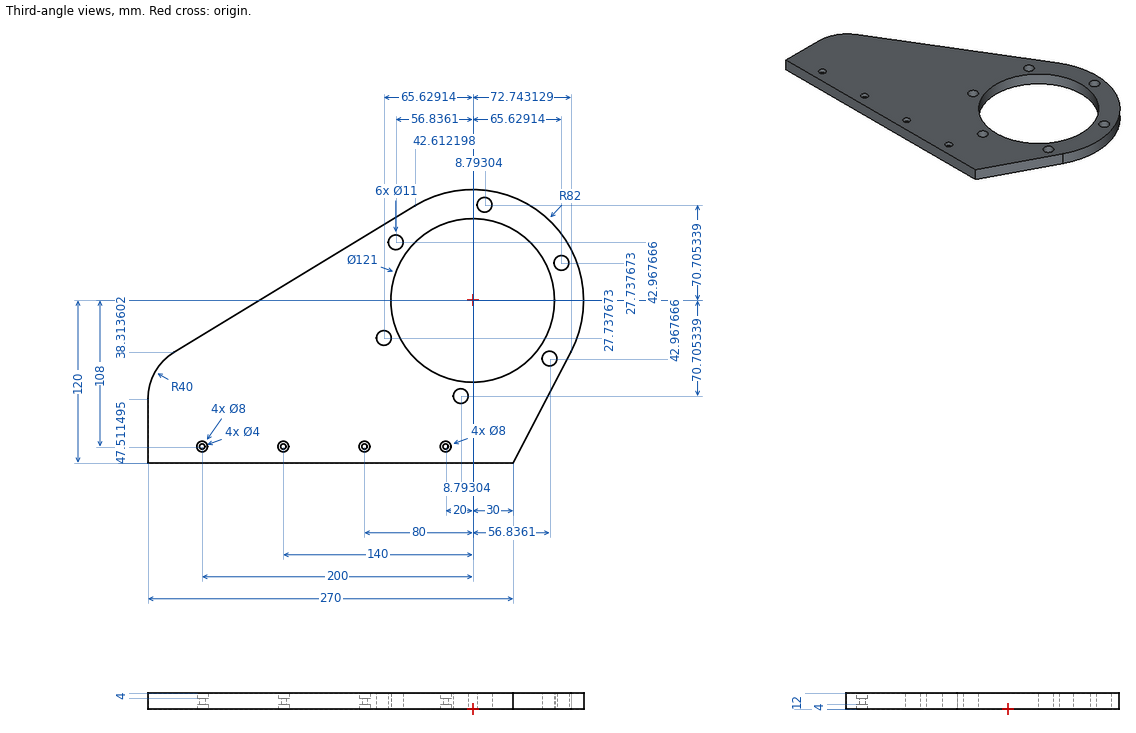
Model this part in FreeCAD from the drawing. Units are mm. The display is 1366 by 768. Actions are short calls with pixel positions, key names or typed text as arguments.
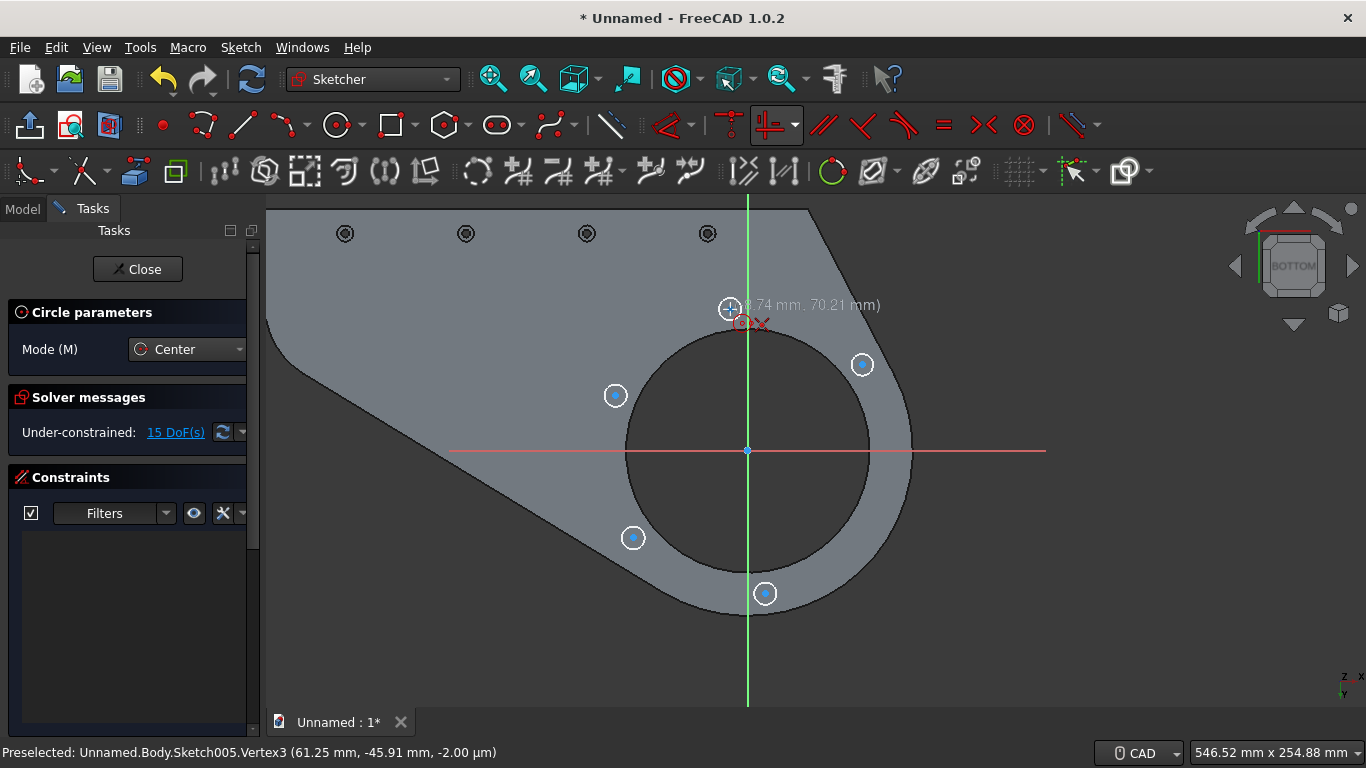
scroll(880, 507, up, 4)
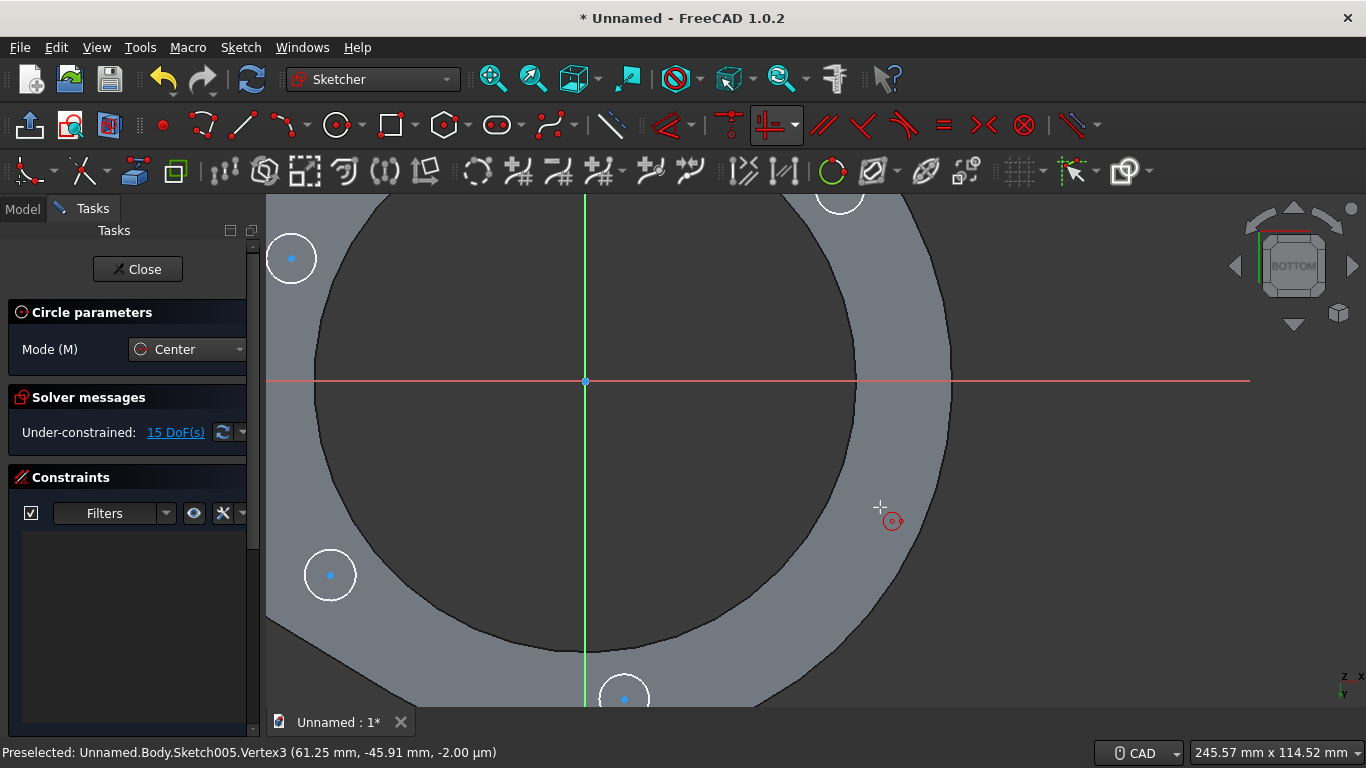
click(879, 506)
click(897, 488)
key(Escape)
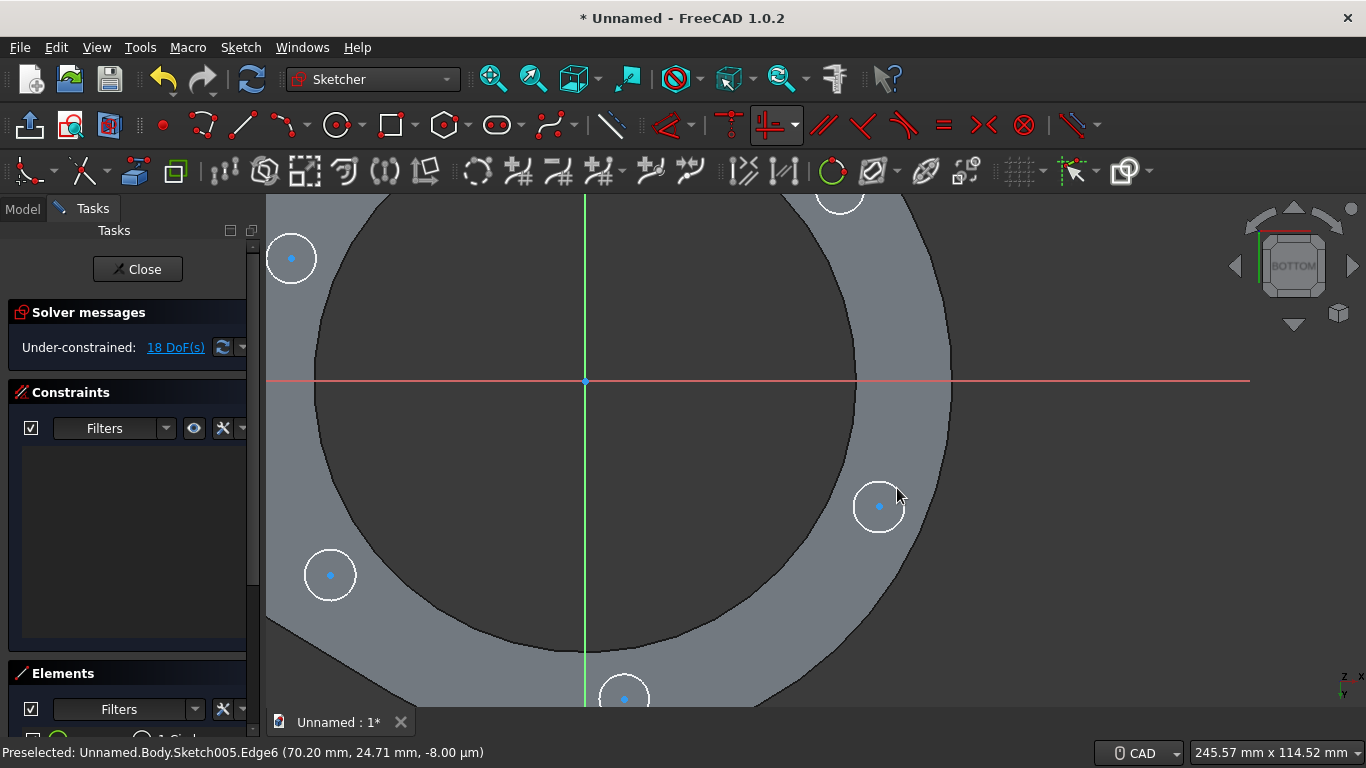
click(348, 557)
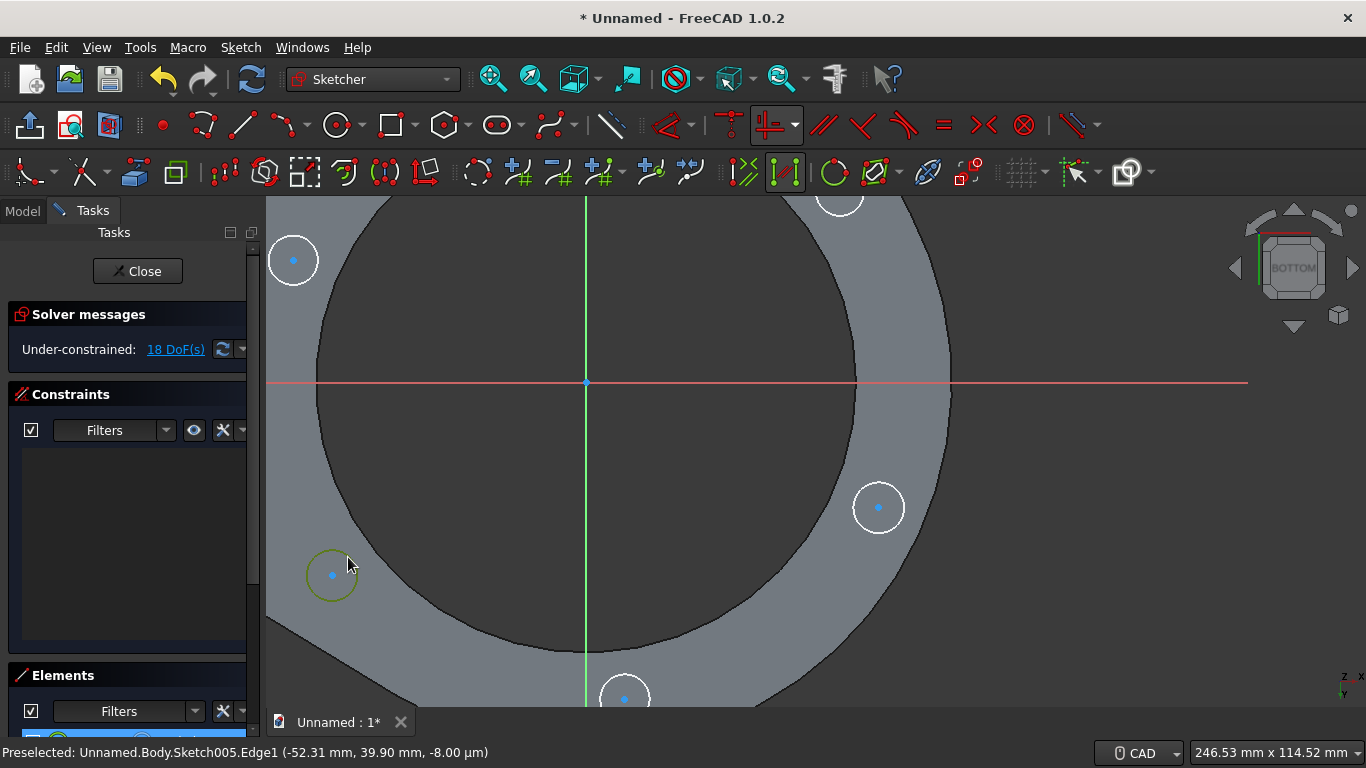
click(626, 674)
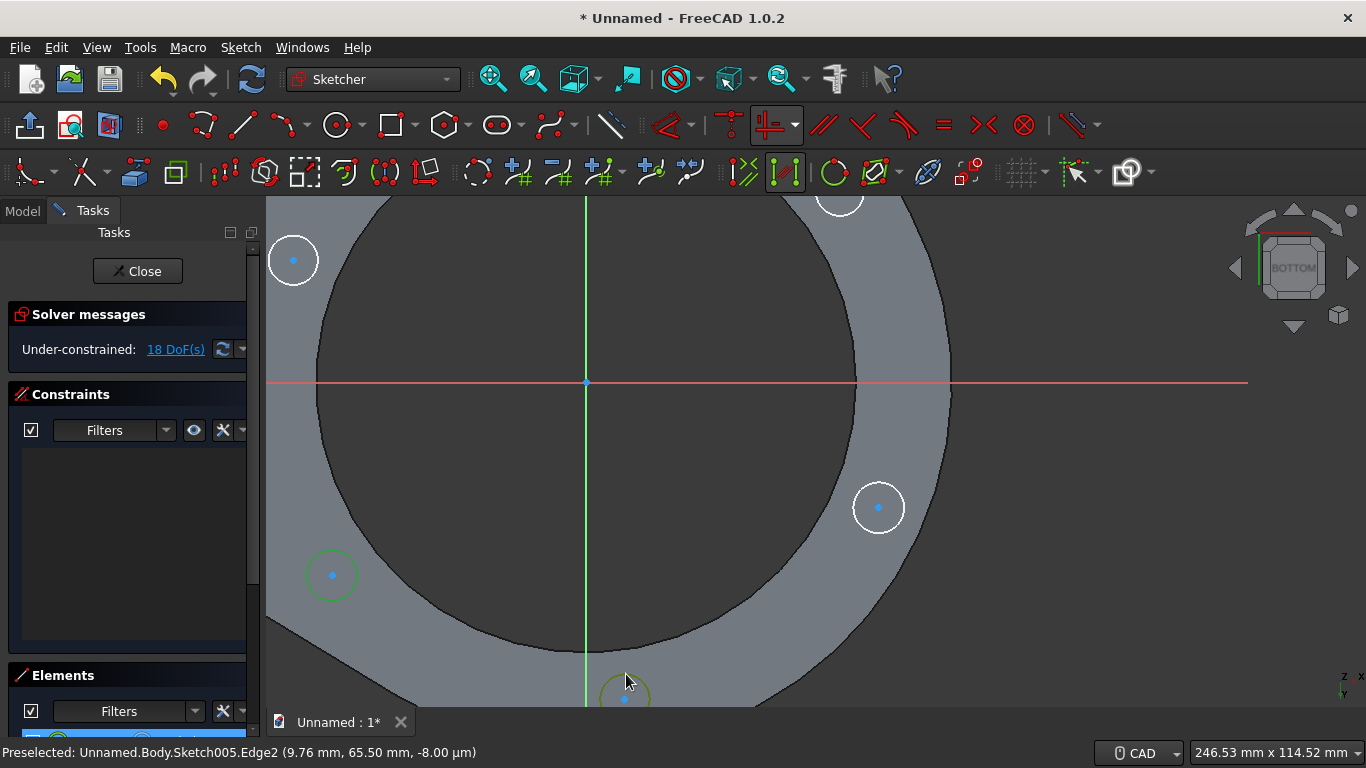
click(311, 243)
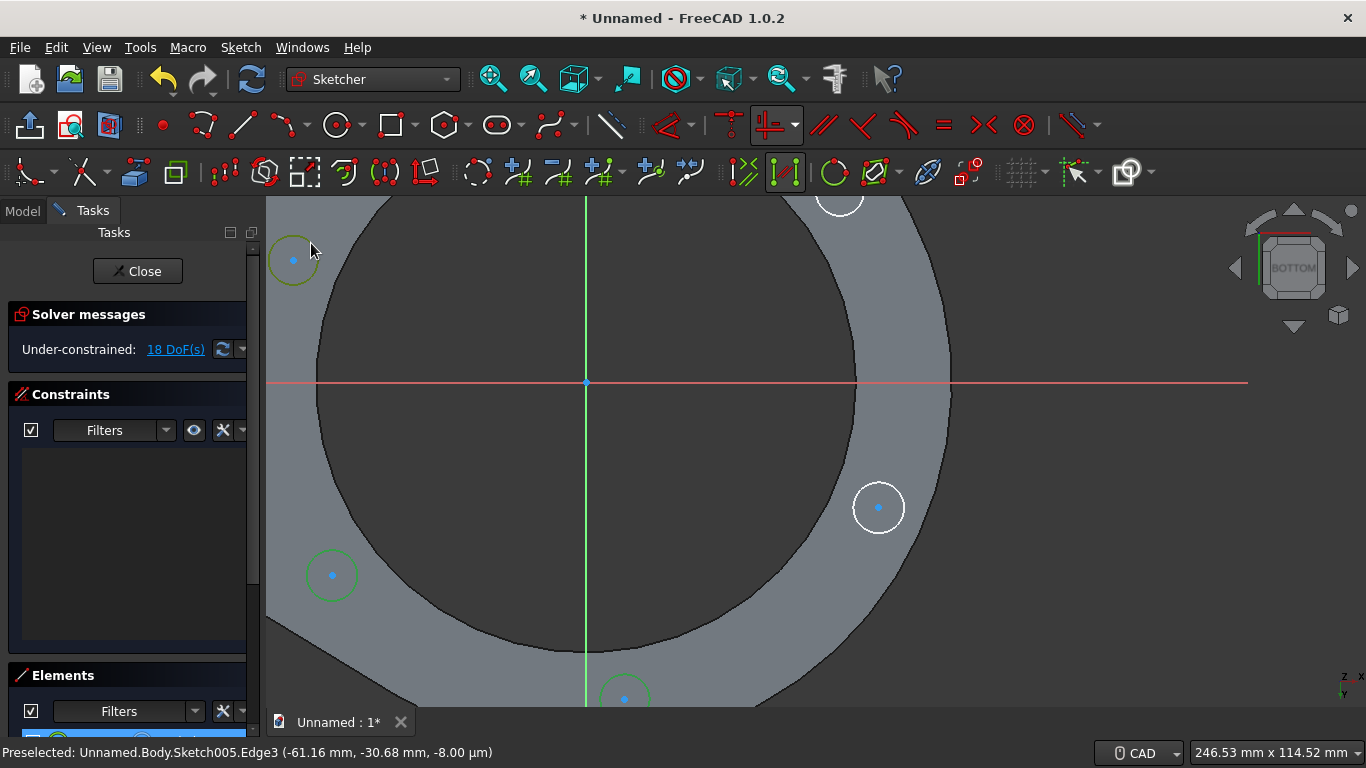
scroll(879, 508, down, 4)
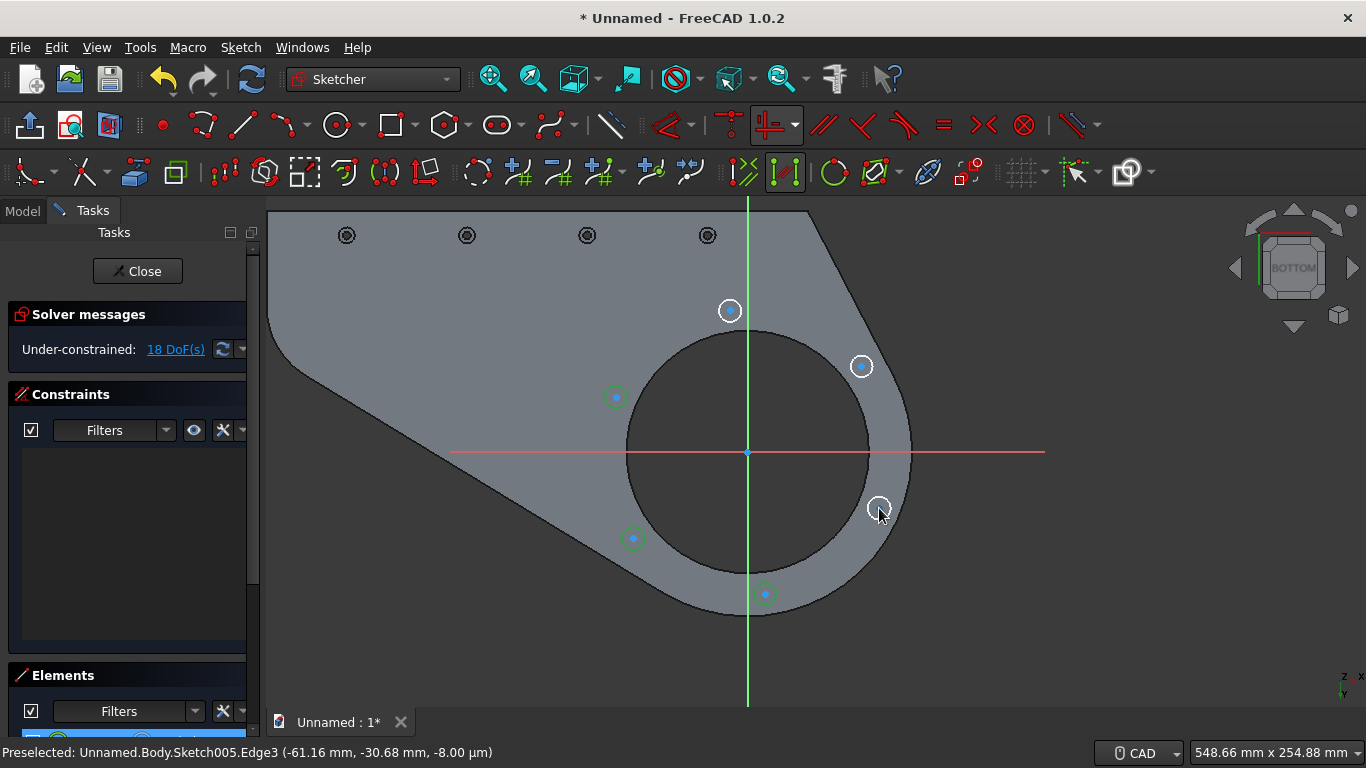
scroll(738, 303, up, 2)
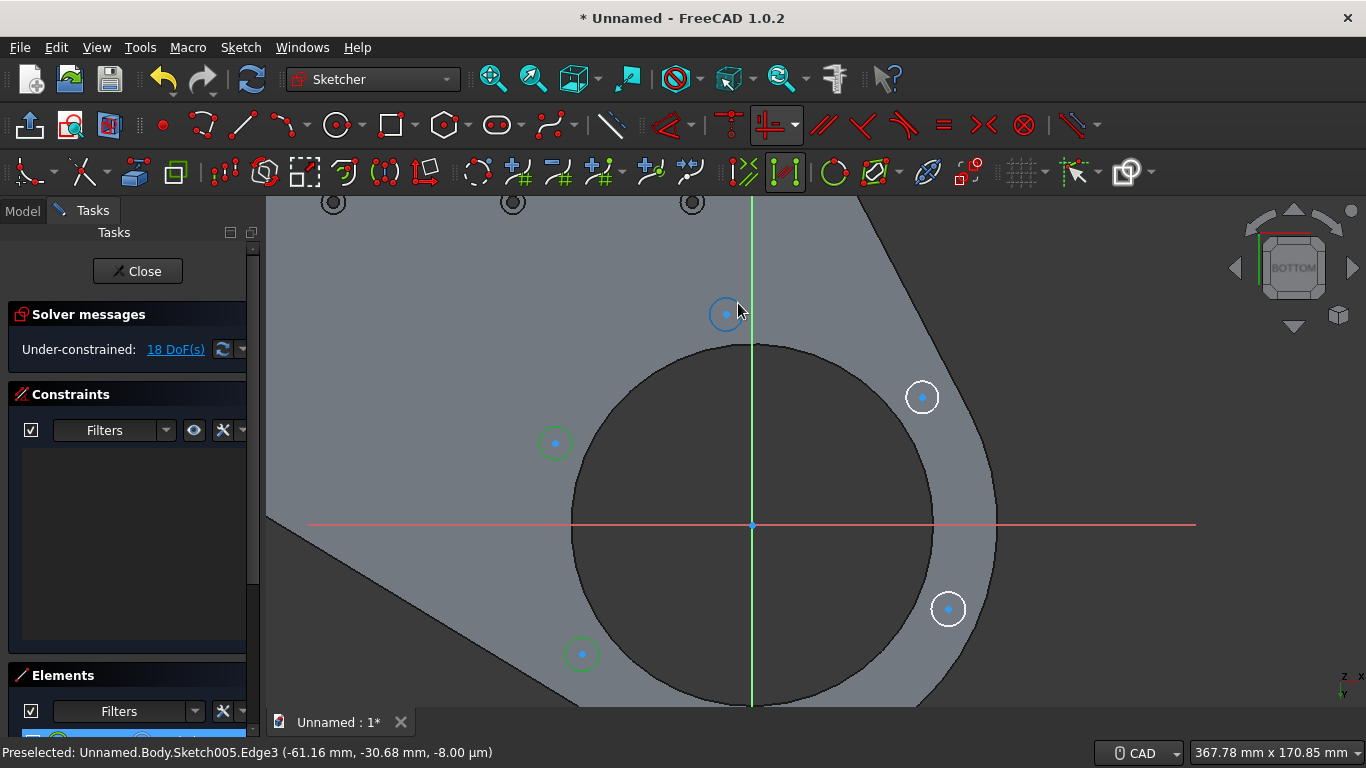
click(738, 303)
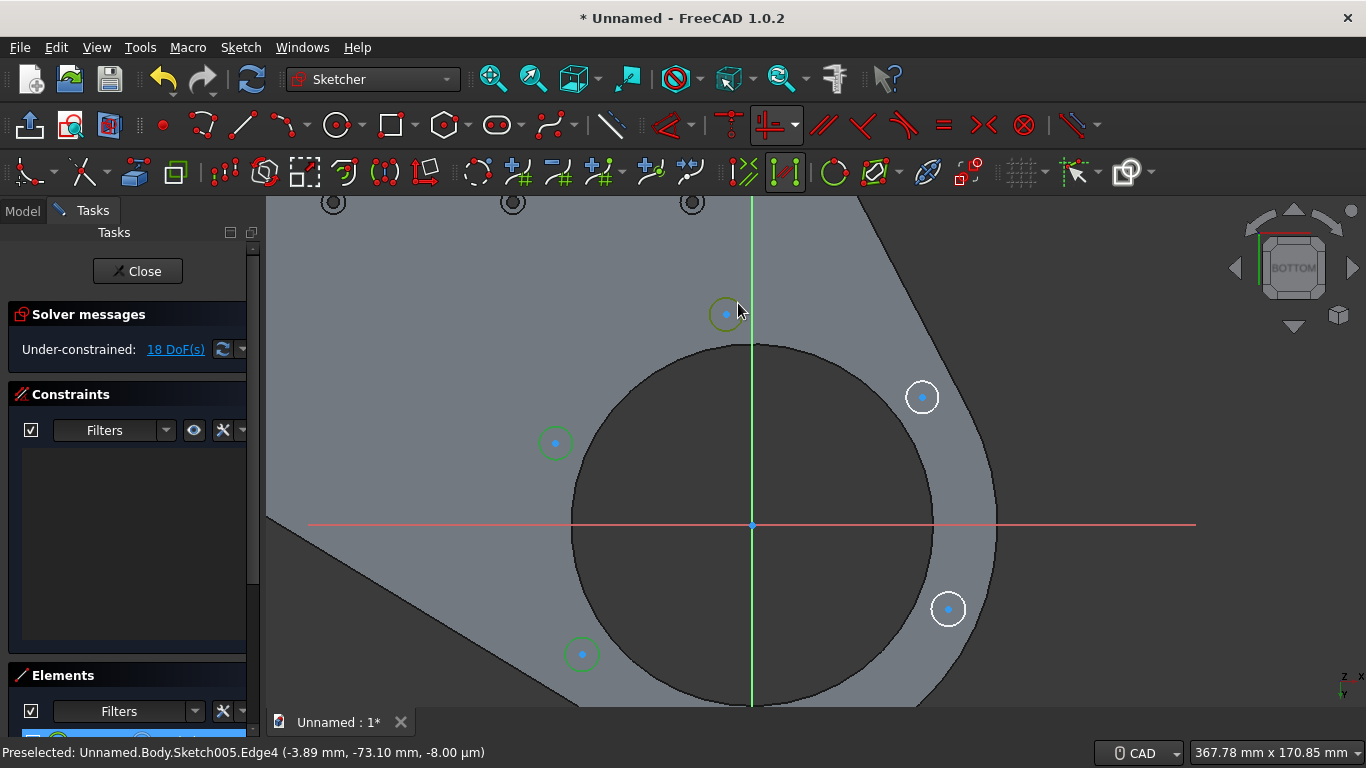
click(934, 386)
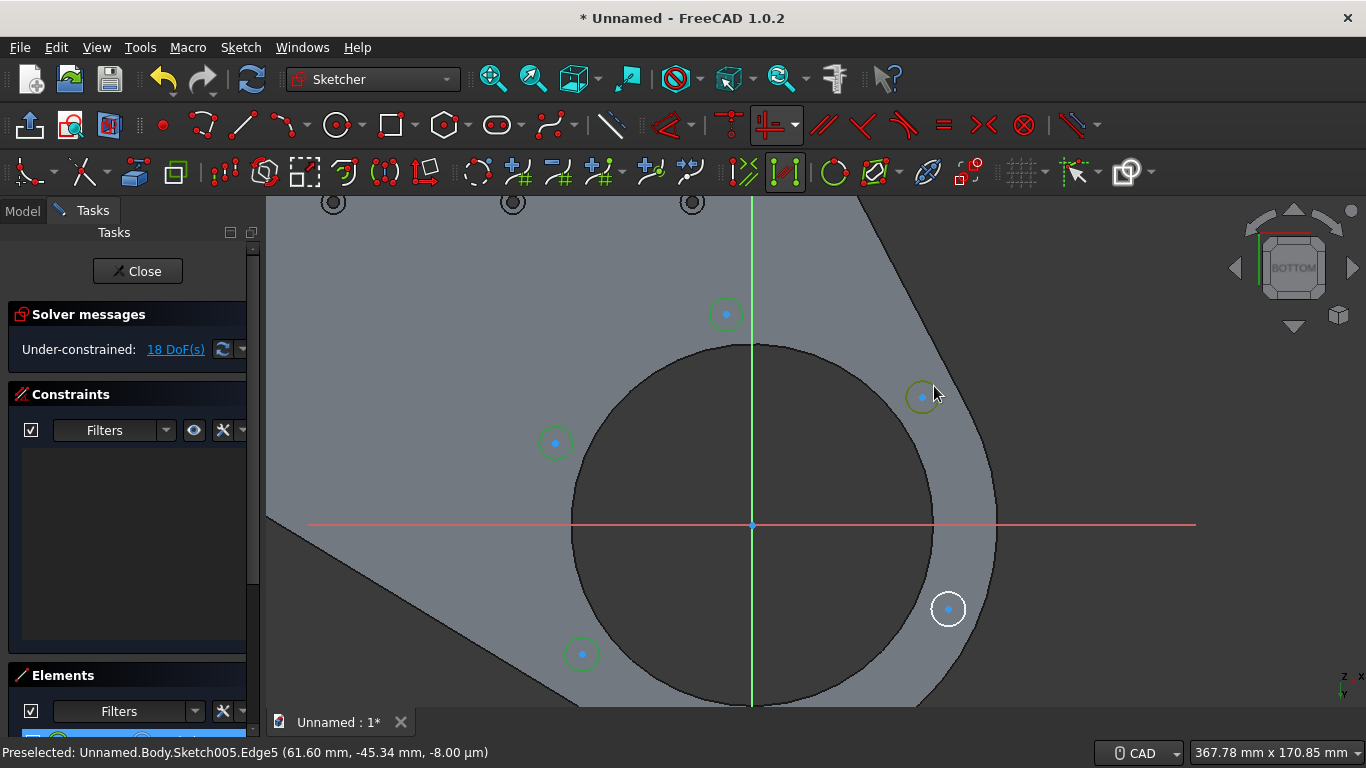
click(960, 597)